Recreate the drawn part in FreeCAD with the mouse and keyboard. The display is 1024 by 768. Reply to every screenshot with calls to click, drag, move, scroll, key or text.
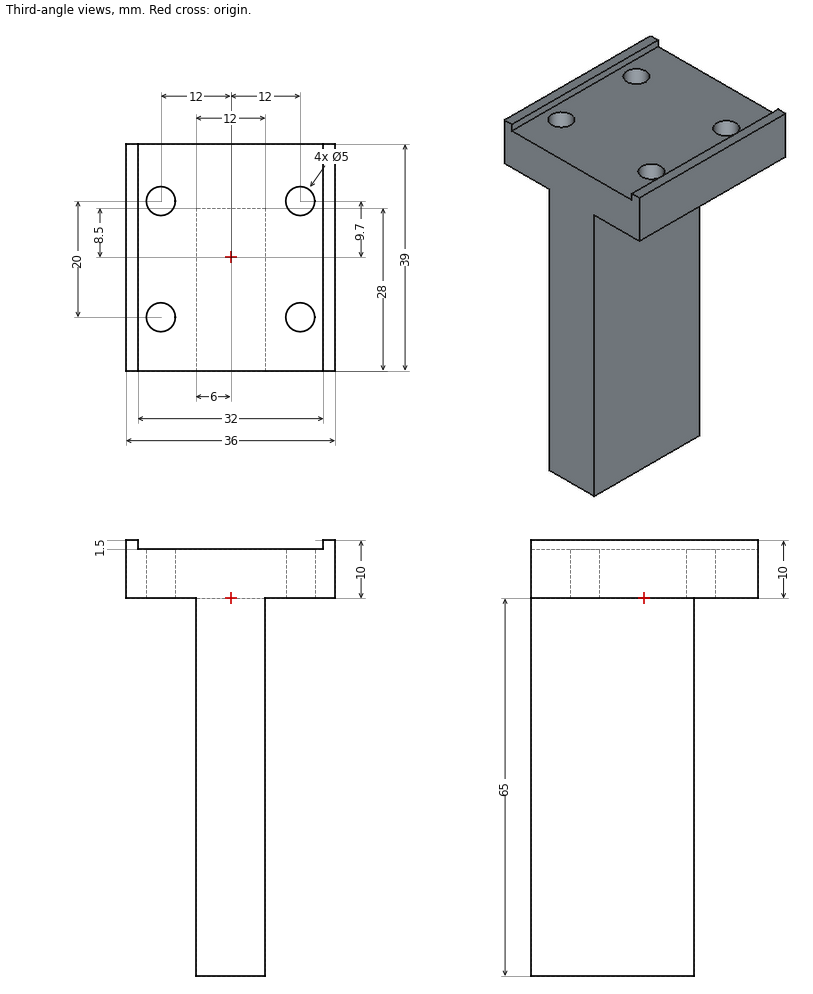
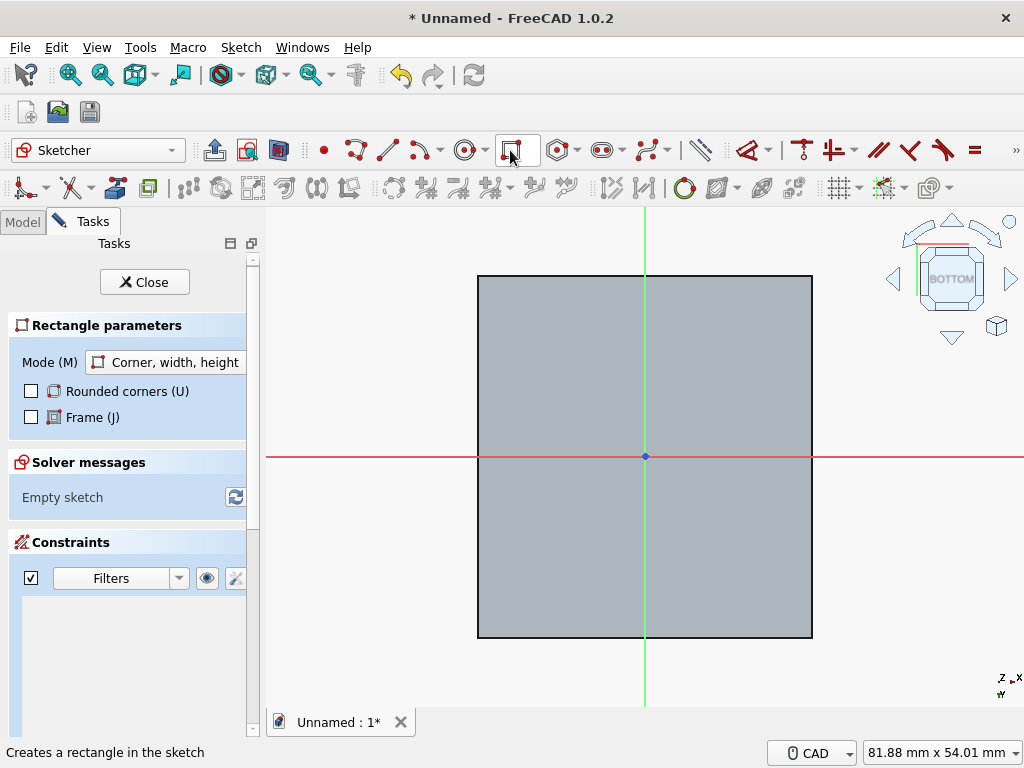
click(589, 276)
move(701, 536)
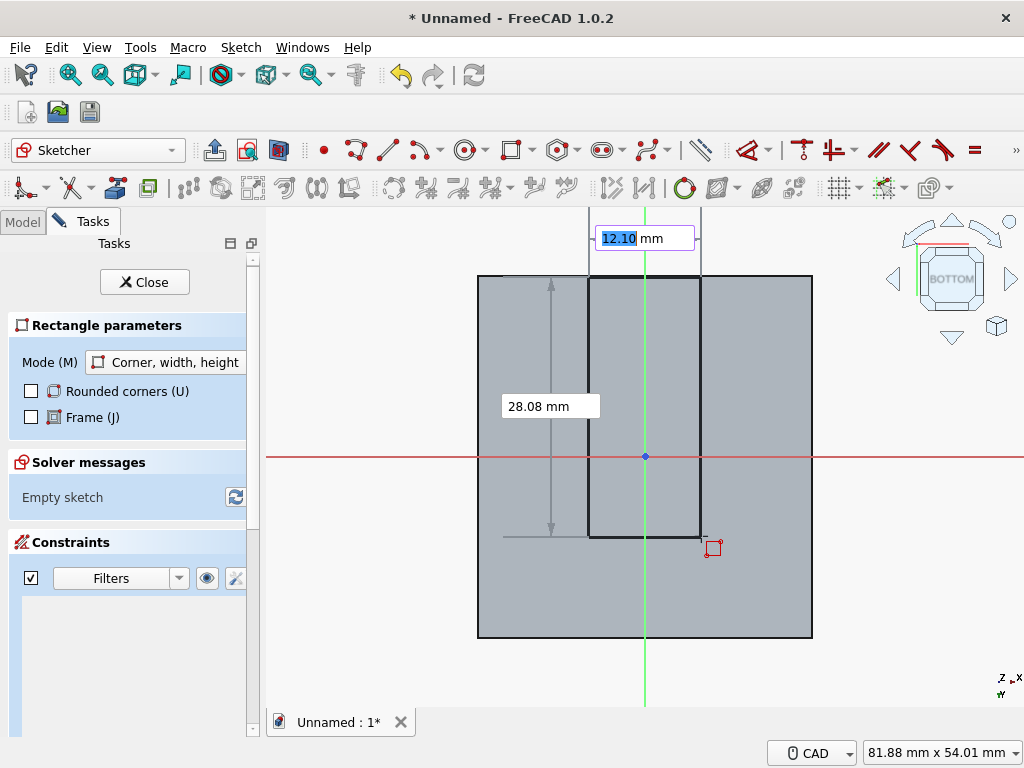
text(12)
key(Tab)
text(28)
key(Return)
key(Escape)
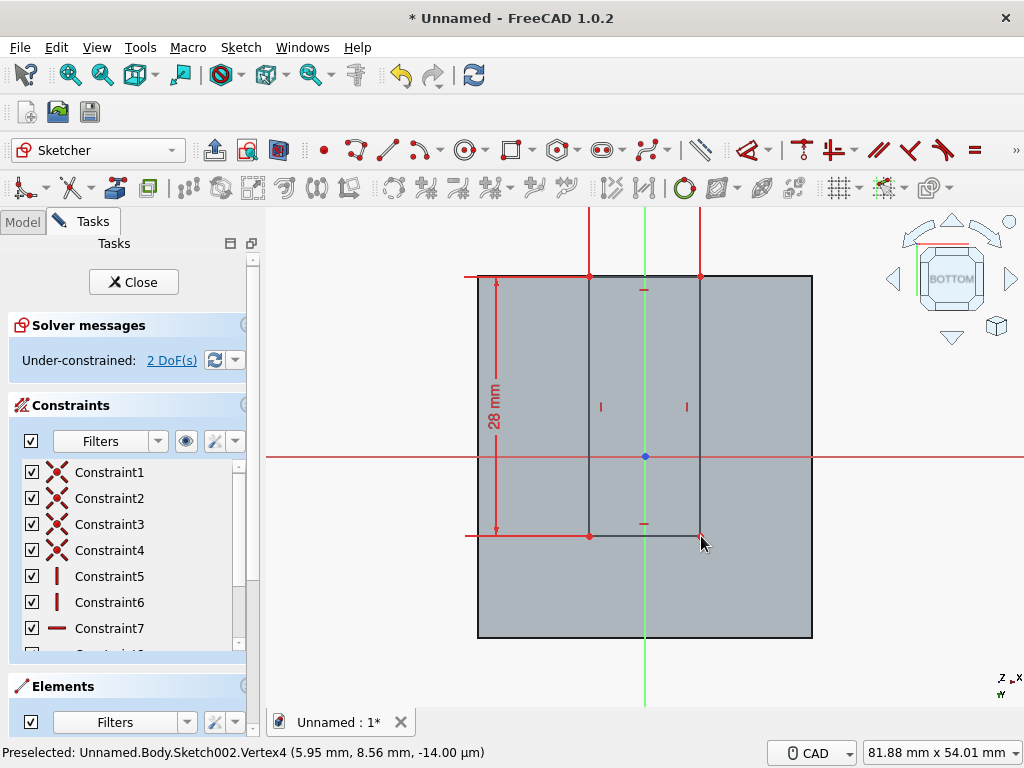
click(748, 150)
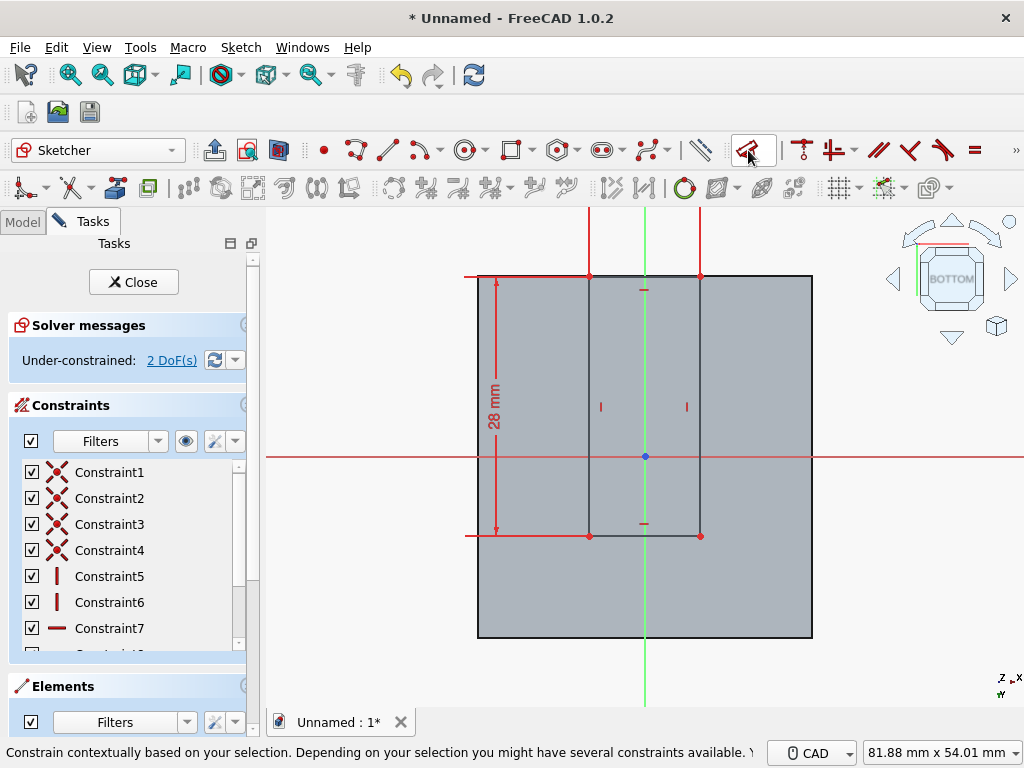
click(589, 277)
click(617, 243)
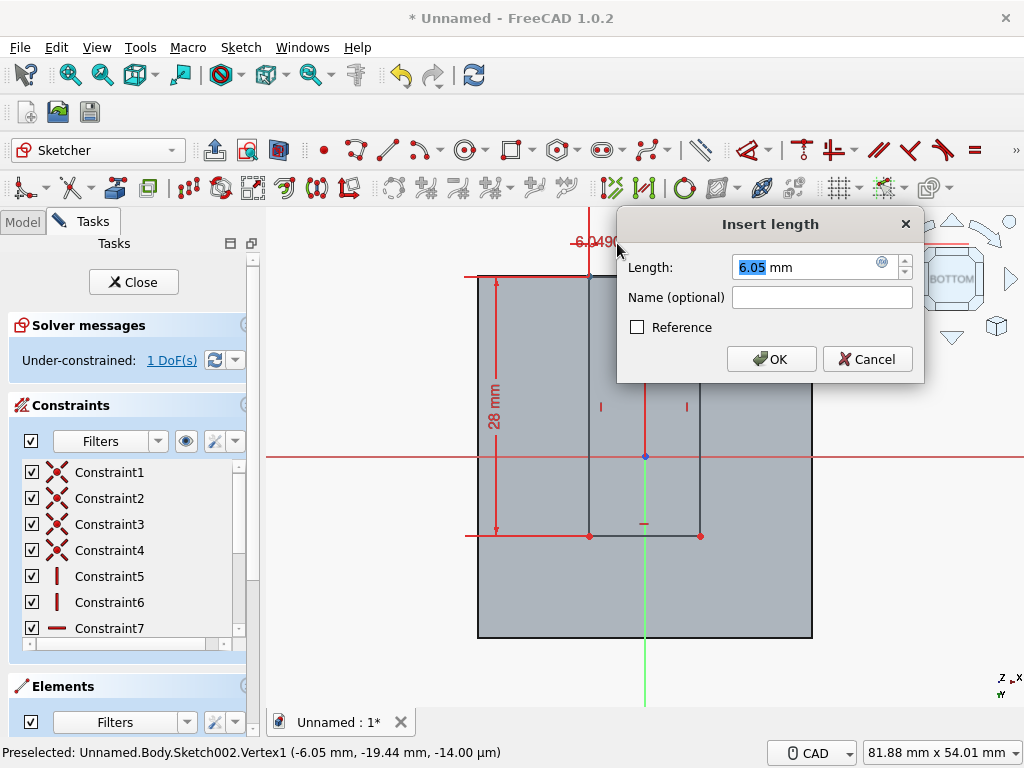
text(6)
key(Return)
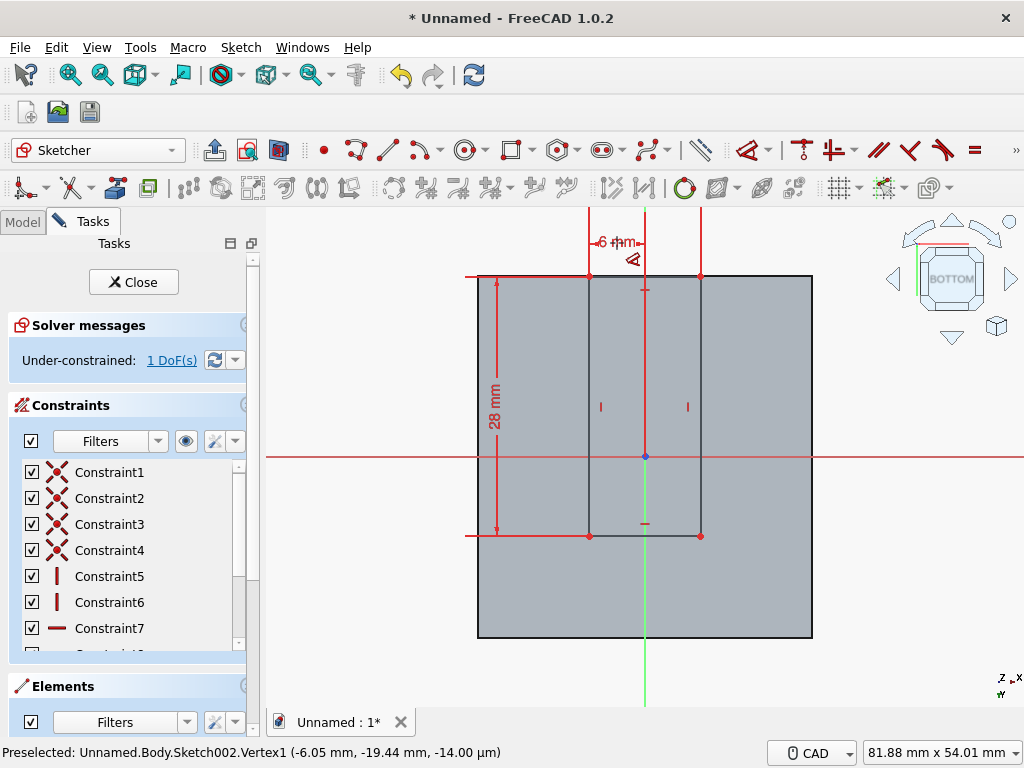
click(589, 536)
click(555, 497)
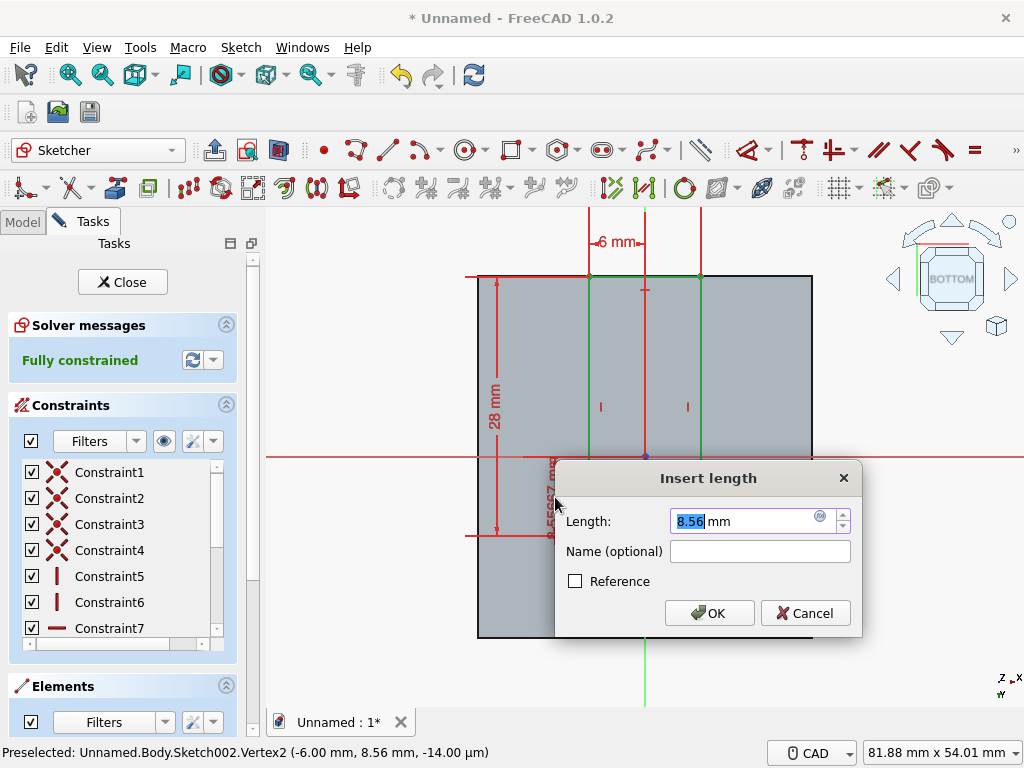
text(8.5)
key(Return)
key(Escape)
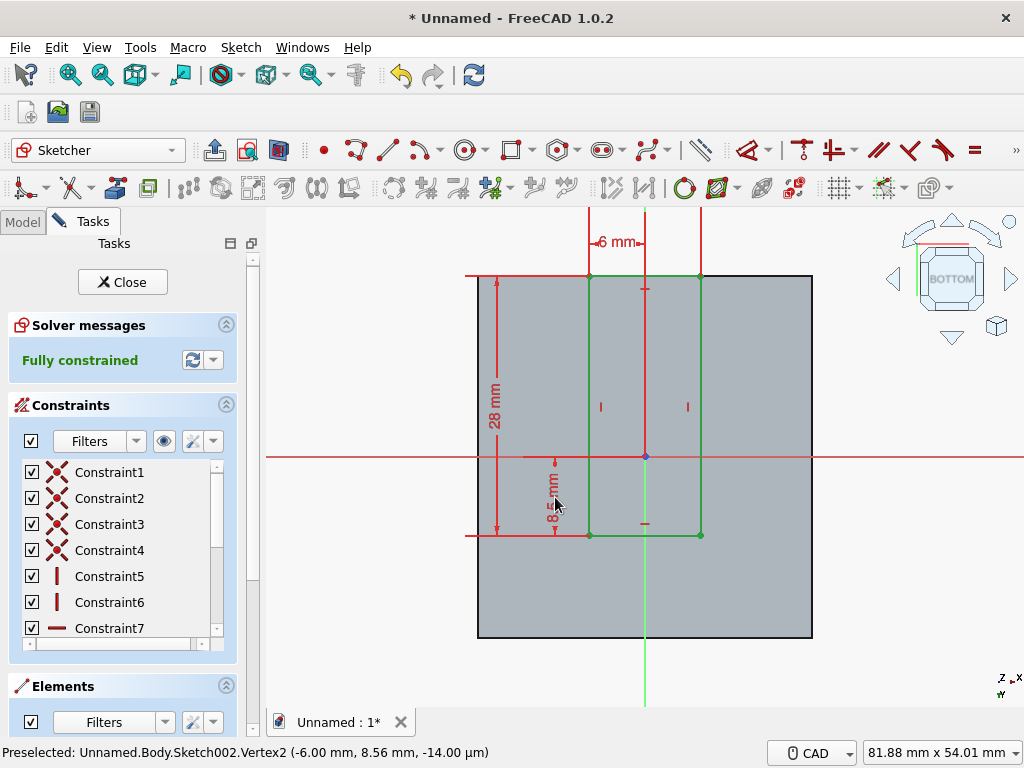
click(123, 282)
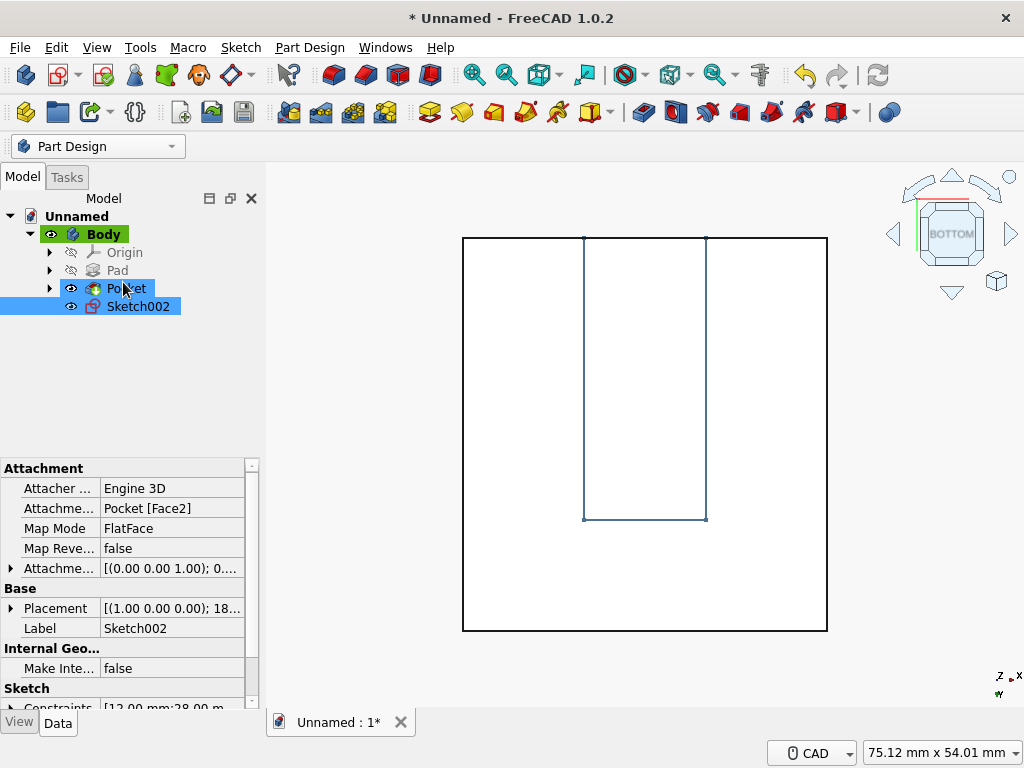
click(430, 112)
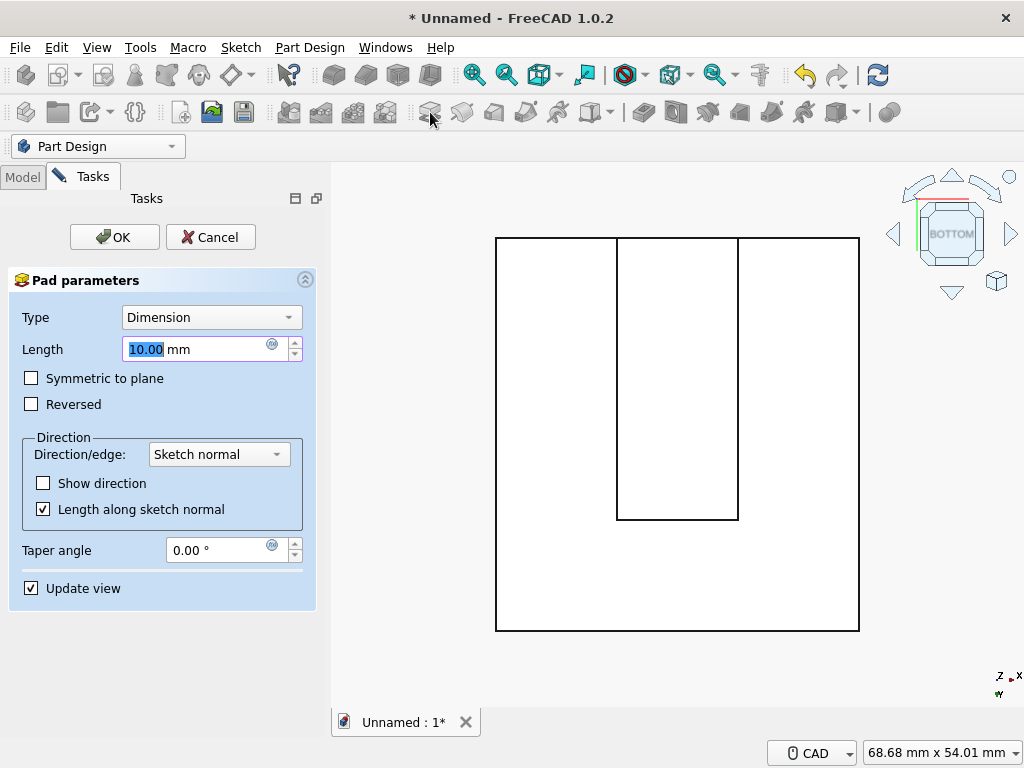
text(65)
key(Tab)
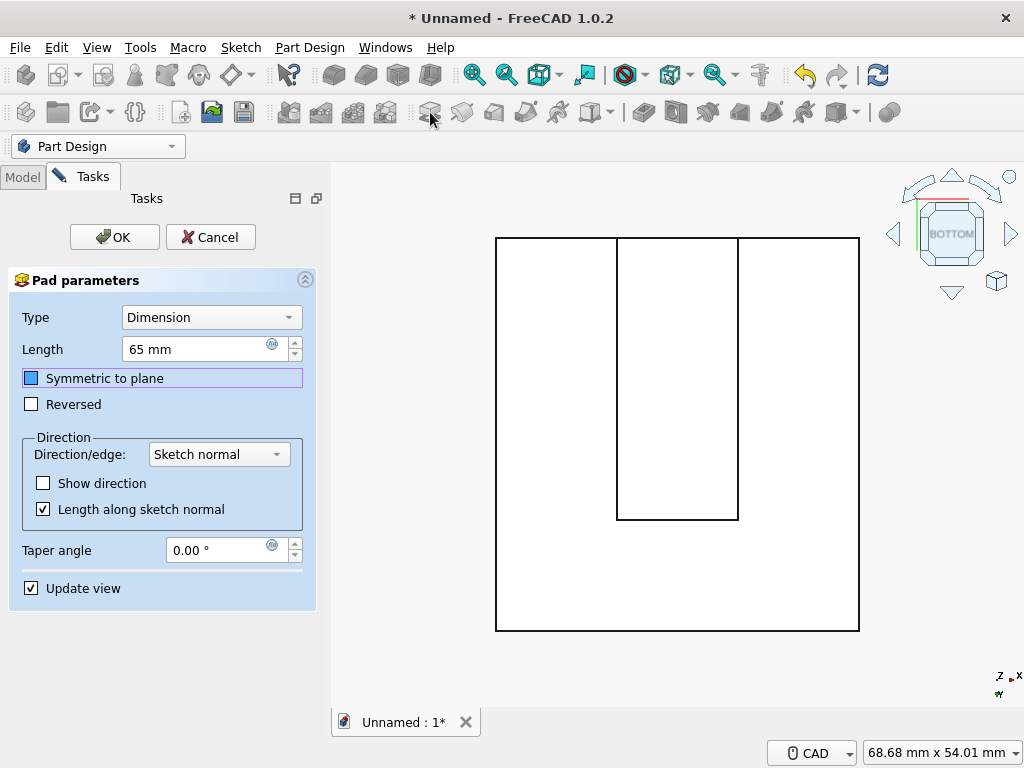
click(115, 237)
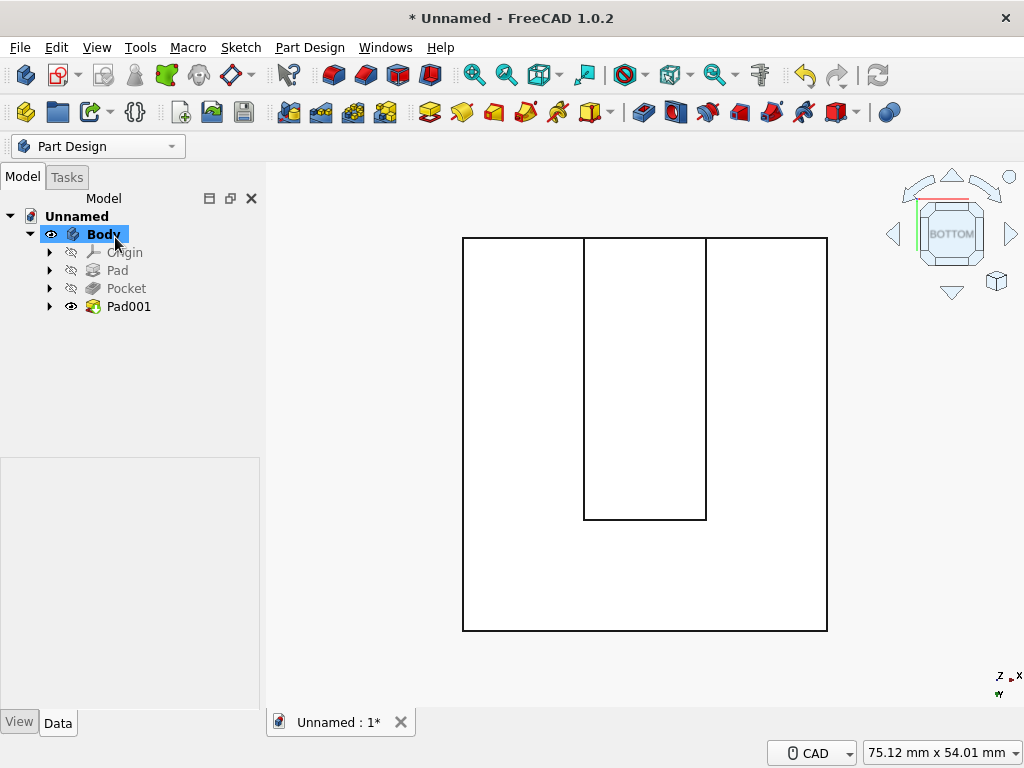
click(749, 546)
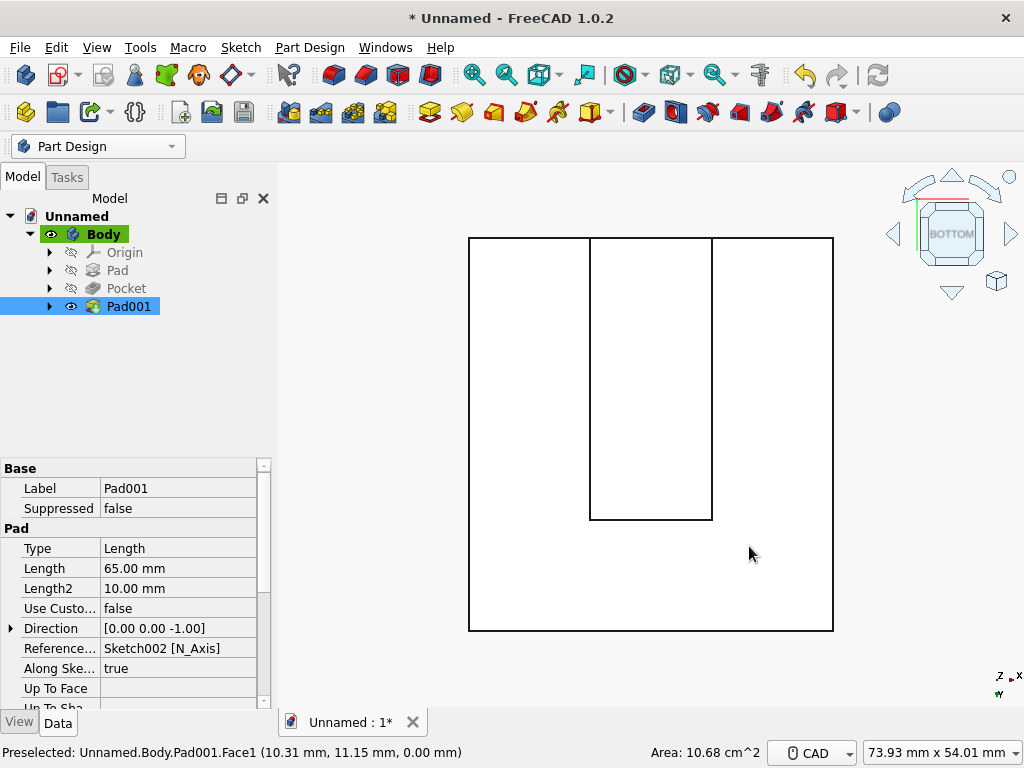
click(58, 76)